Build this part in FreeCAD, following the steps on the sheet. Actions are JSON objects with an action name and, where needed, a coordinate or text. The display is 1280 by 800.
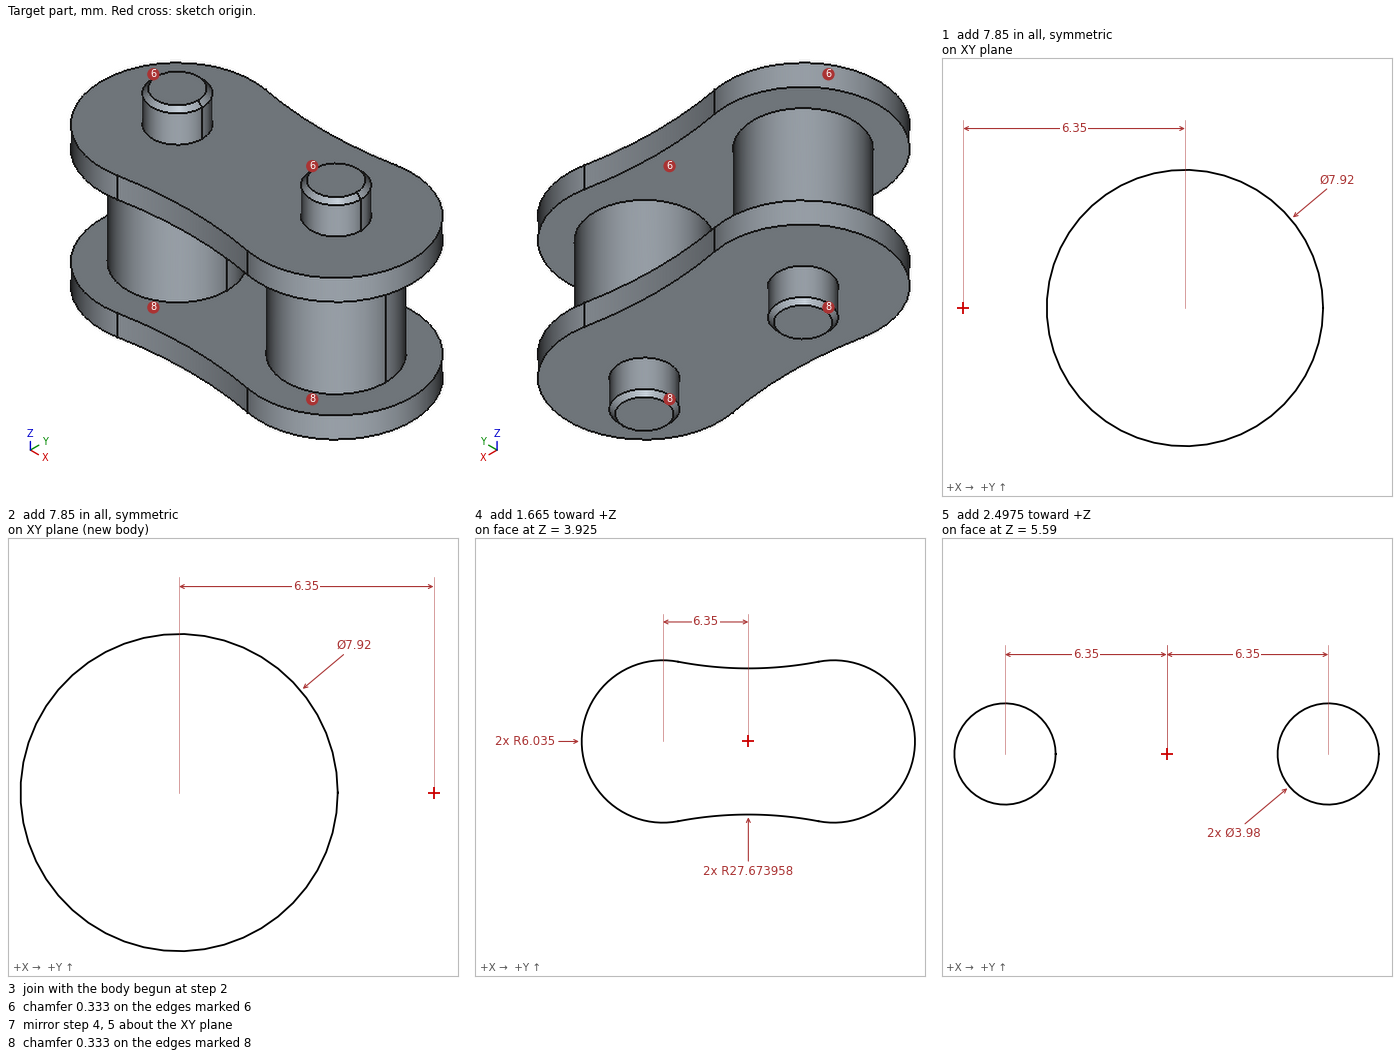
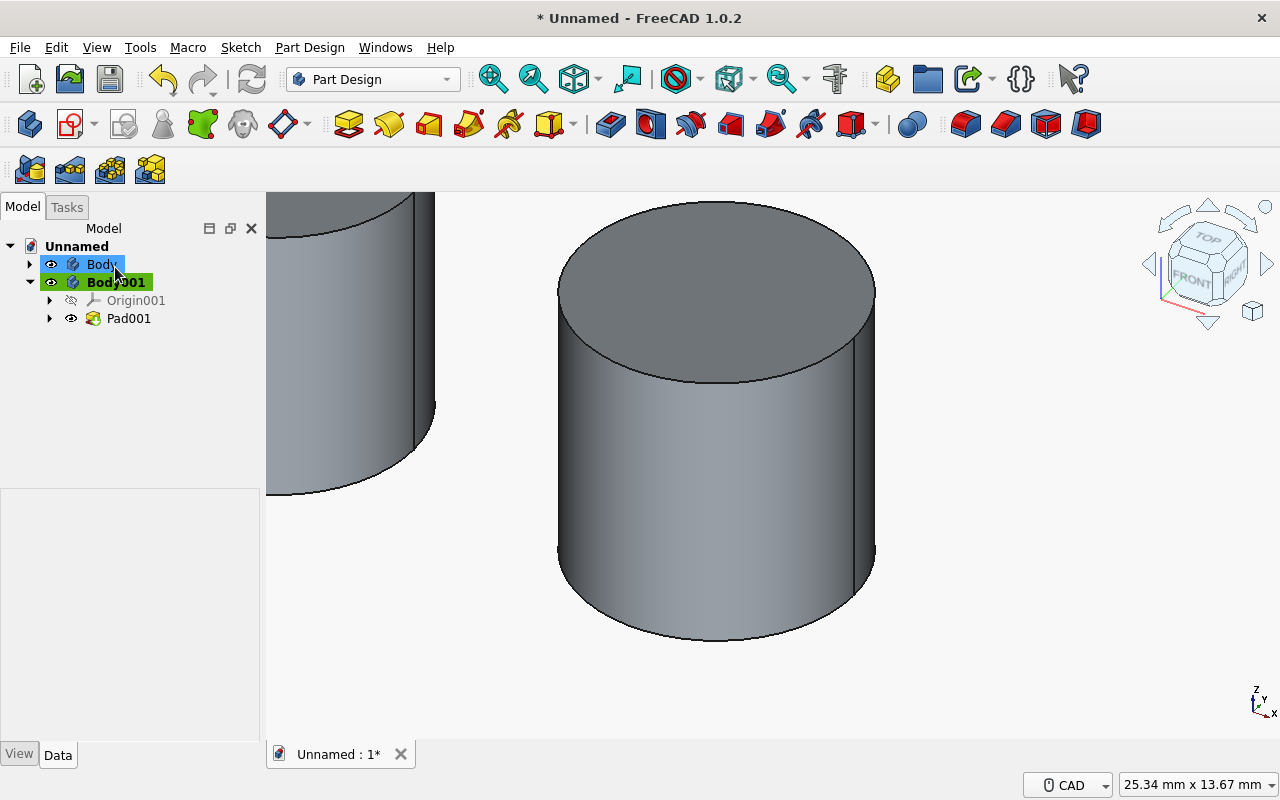
{"action": "key", "text": "v f"}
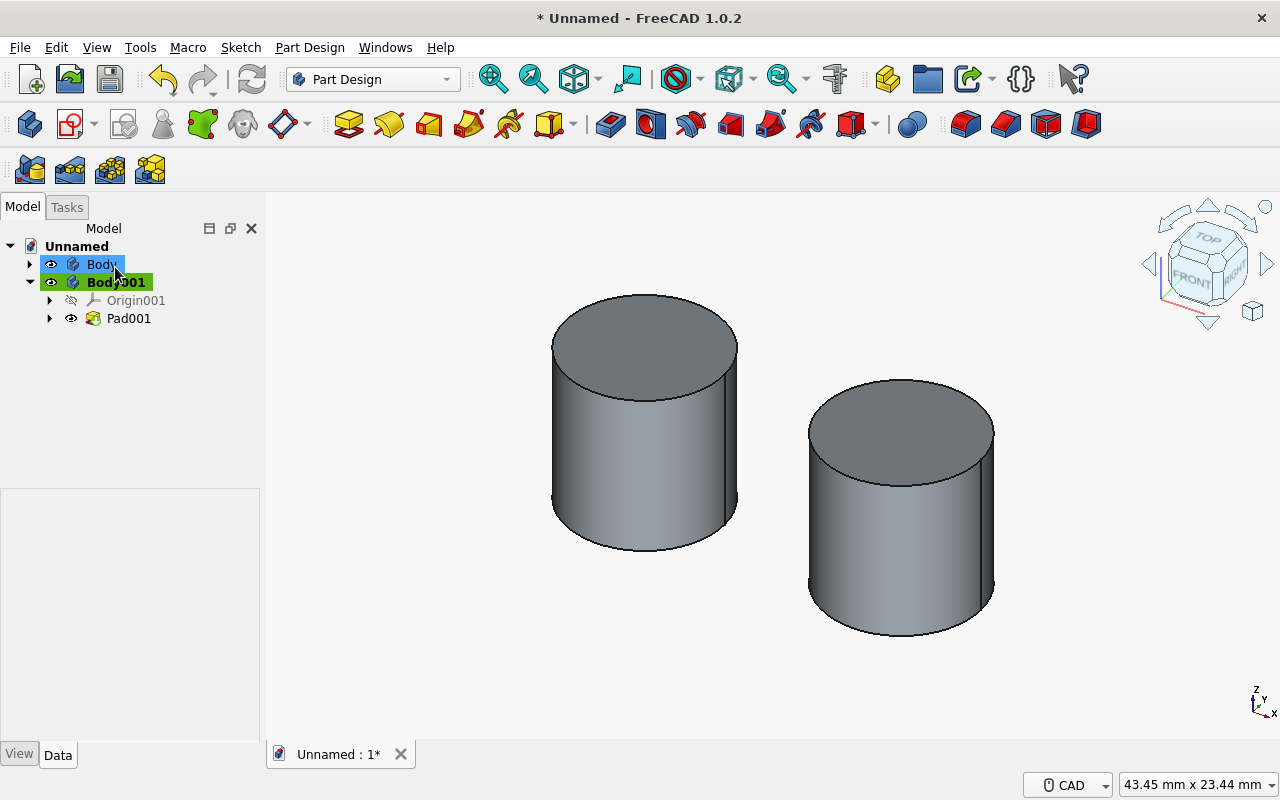
{"action": "double_click", "coordinate": [96, 264]}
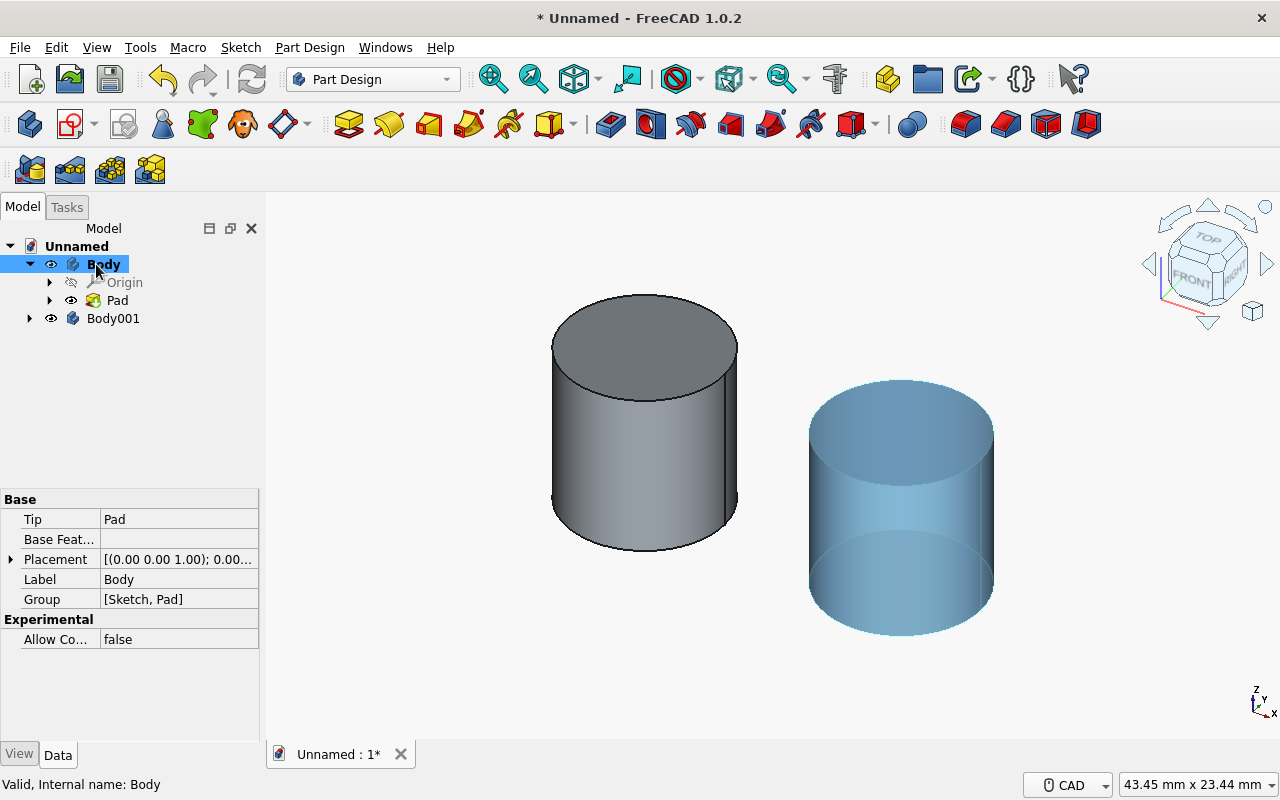
{"action": "left_click", "coordinate": [96, 264]}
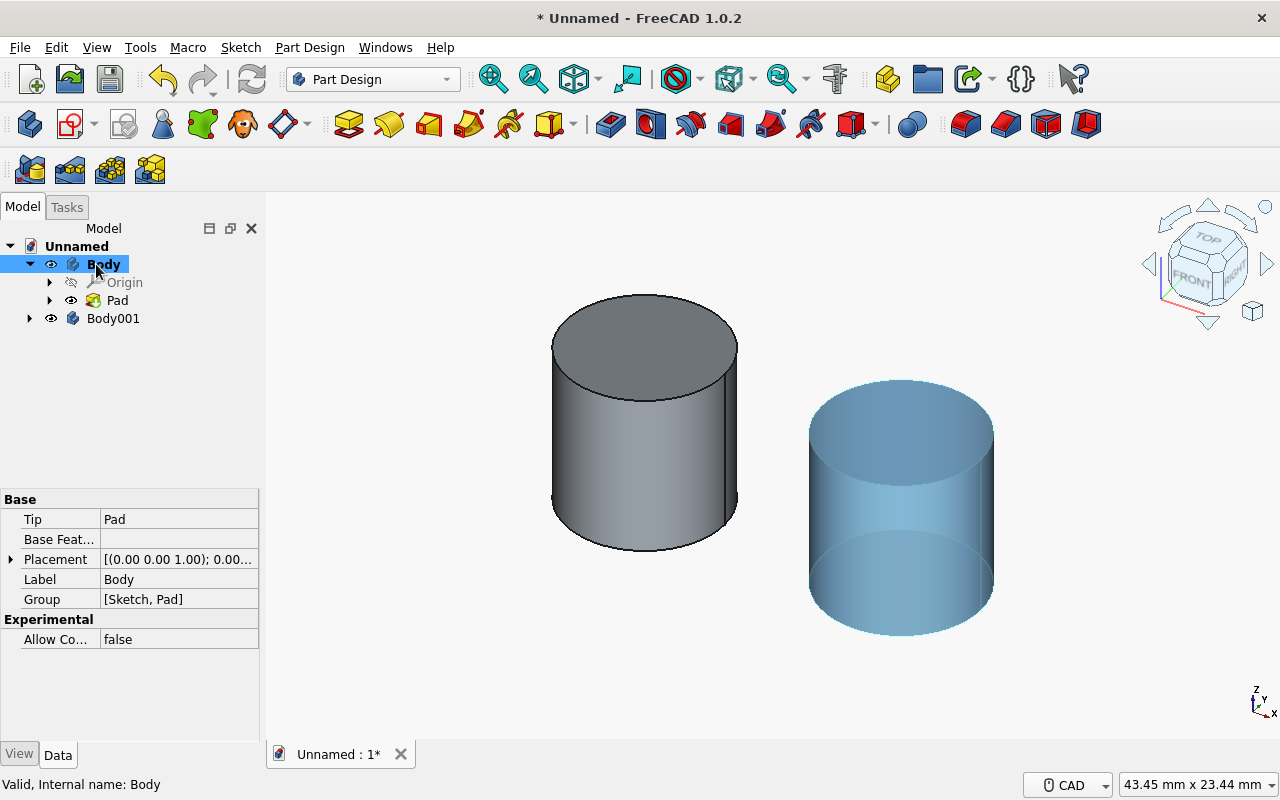
{"action": "left_click", "coordinate": [146, 639]}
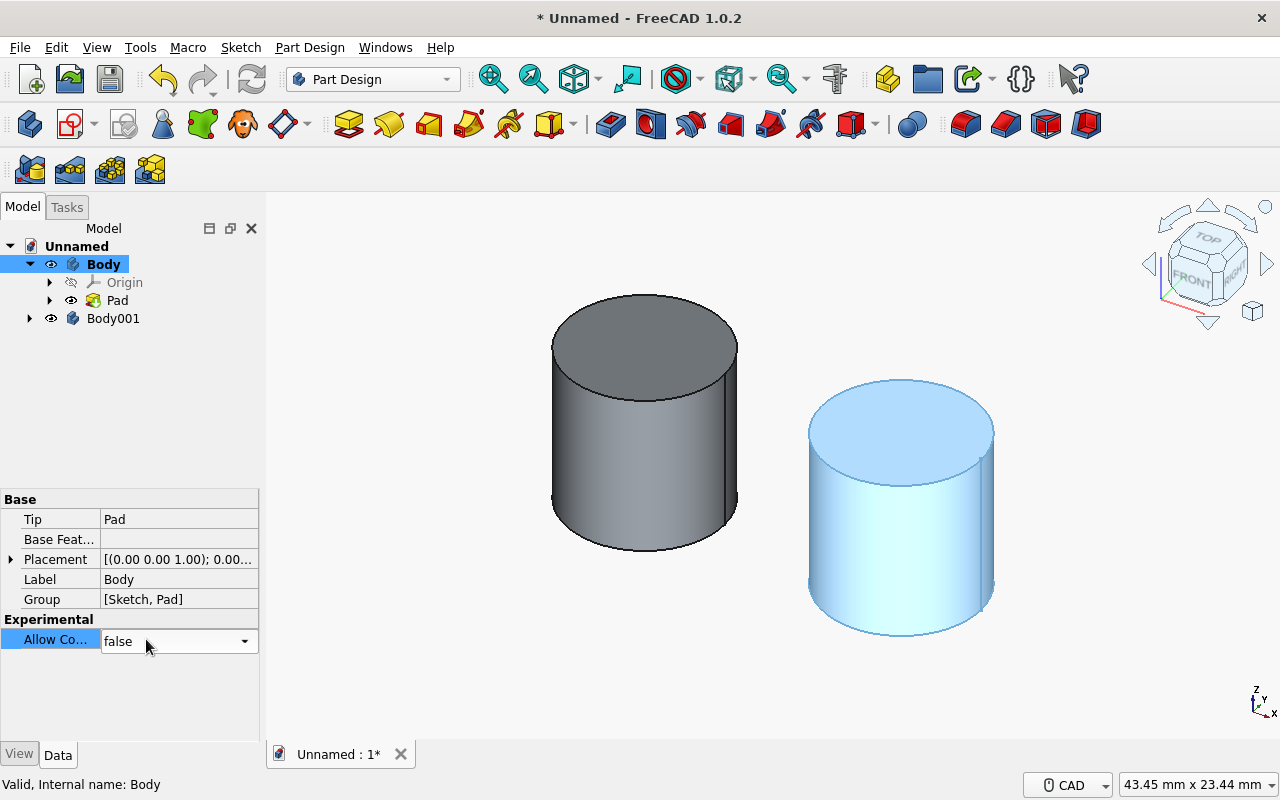
{"action": "left_click", "coordinate": [146, 639]}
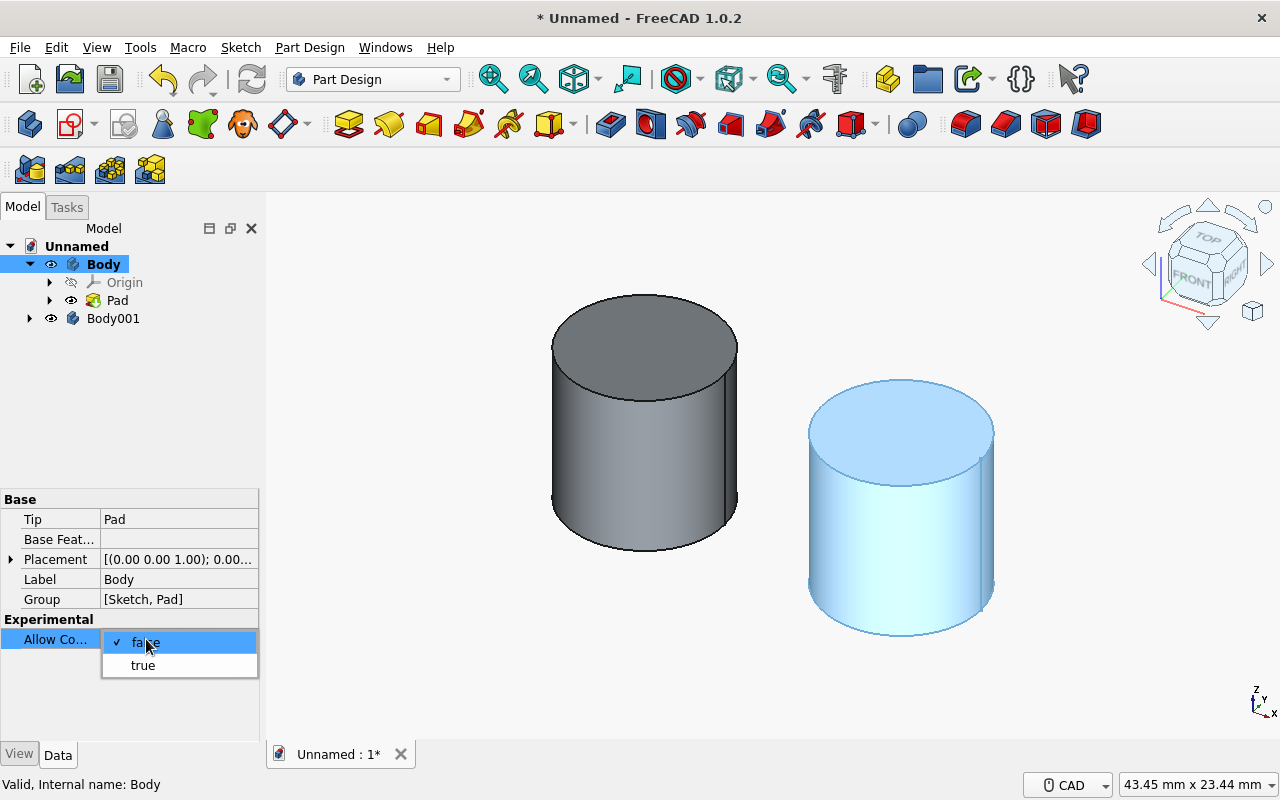
{"action": "left_click", "coordinate": [179, 666]}
{"action": "key", "text": "Return"}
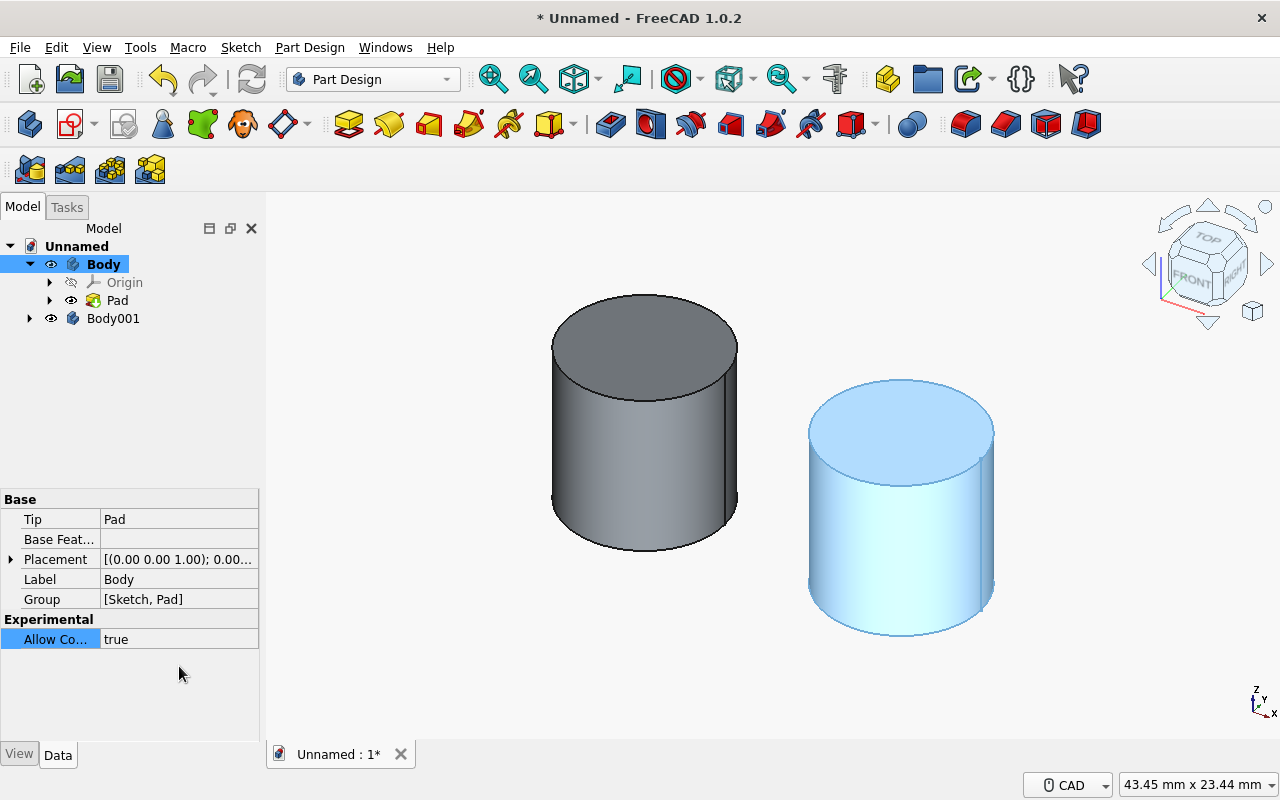
{"action": "left_click", "coordinate": [96, 318]}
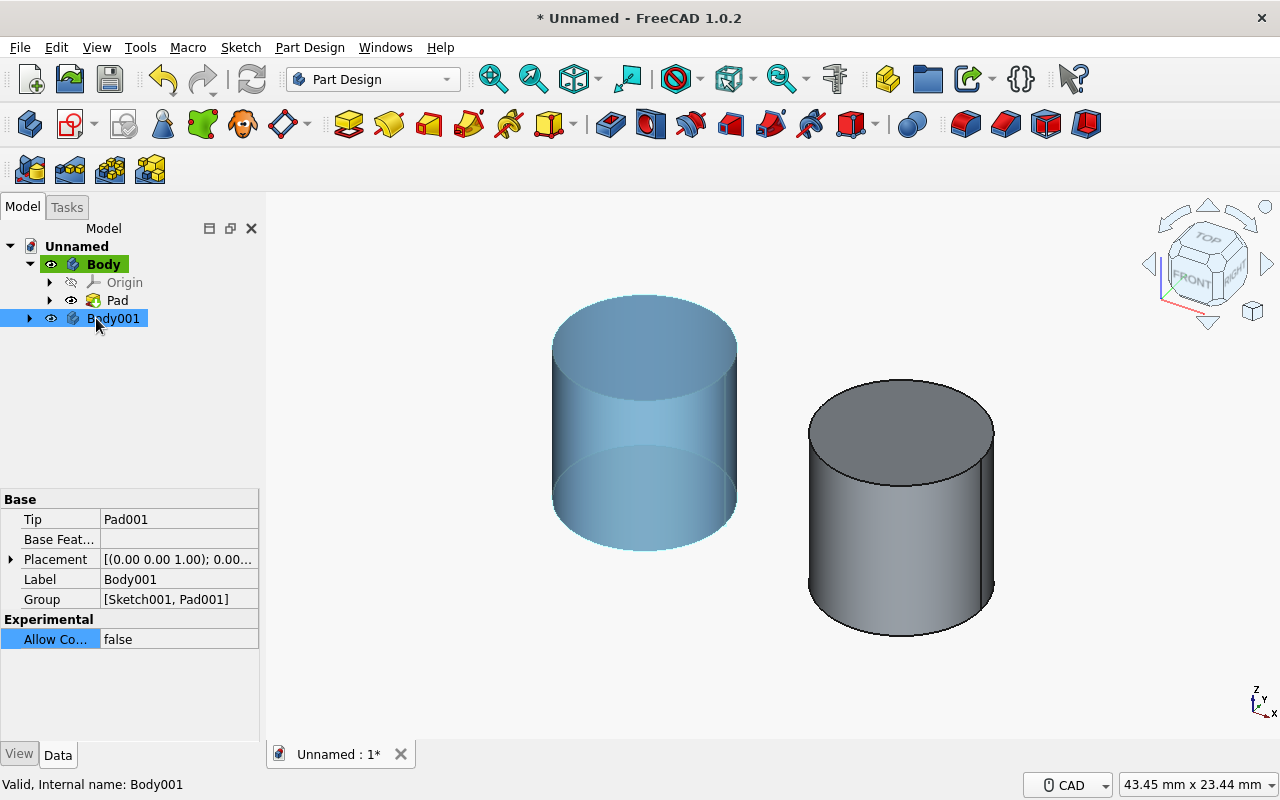
{"action": "left_click", "coordinate": [914, 124]}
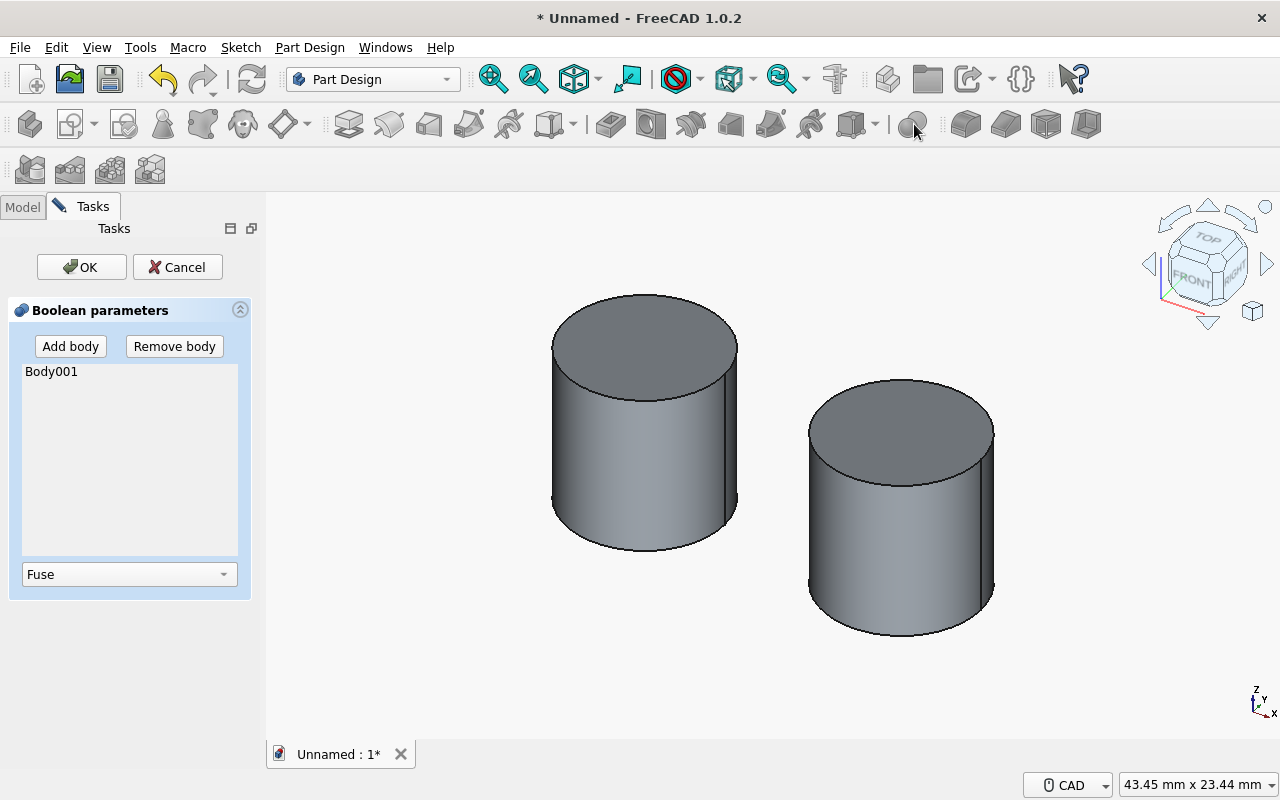
{"action": "left_click", "coordinate": [82, 267]}